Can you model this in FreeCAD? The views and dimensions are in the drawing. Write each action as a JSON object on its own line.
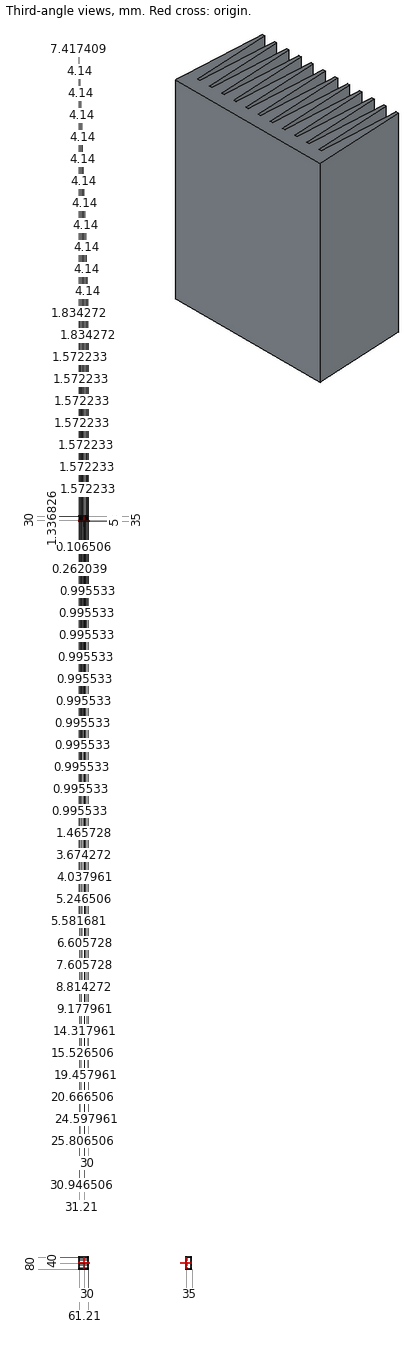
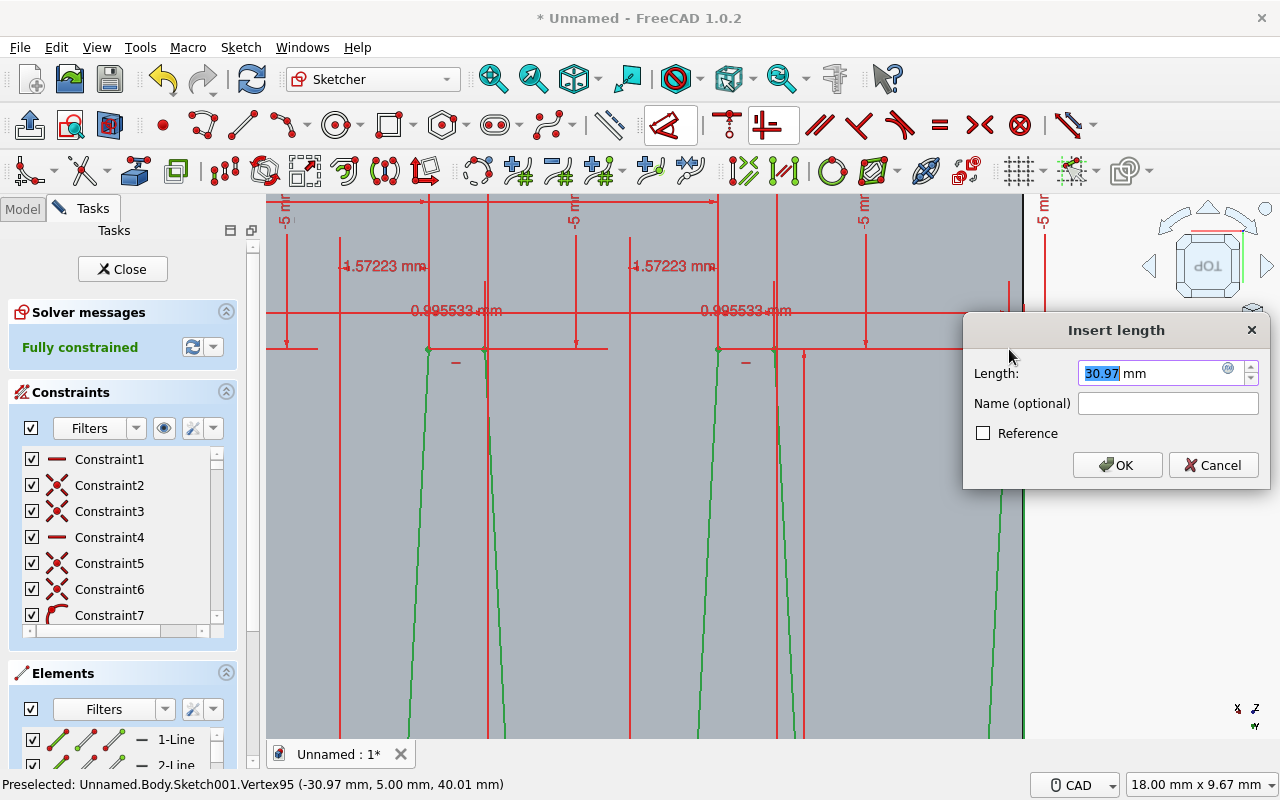
{"action": "type", "text": "30.946506"}
{"action": "key", "text": "Return"}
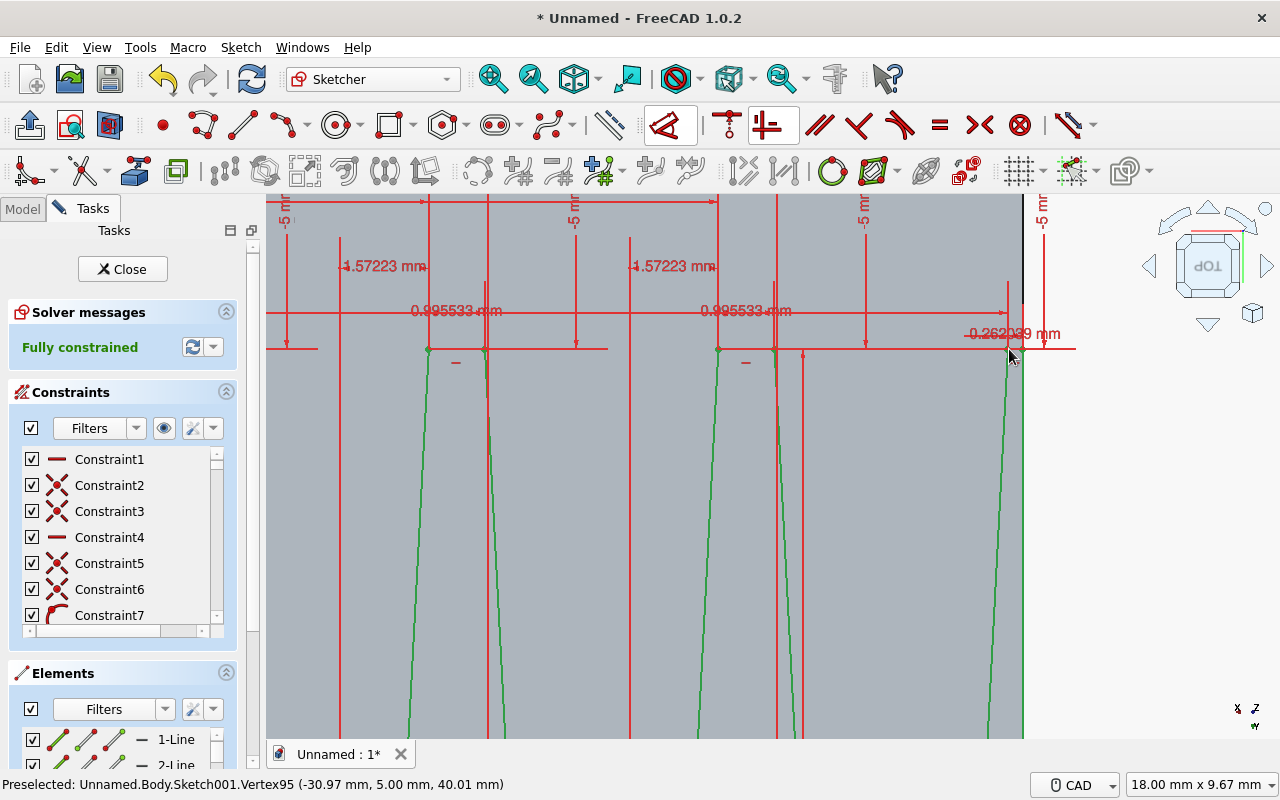
{"action": "left_click", "coordinate": [123, 269]}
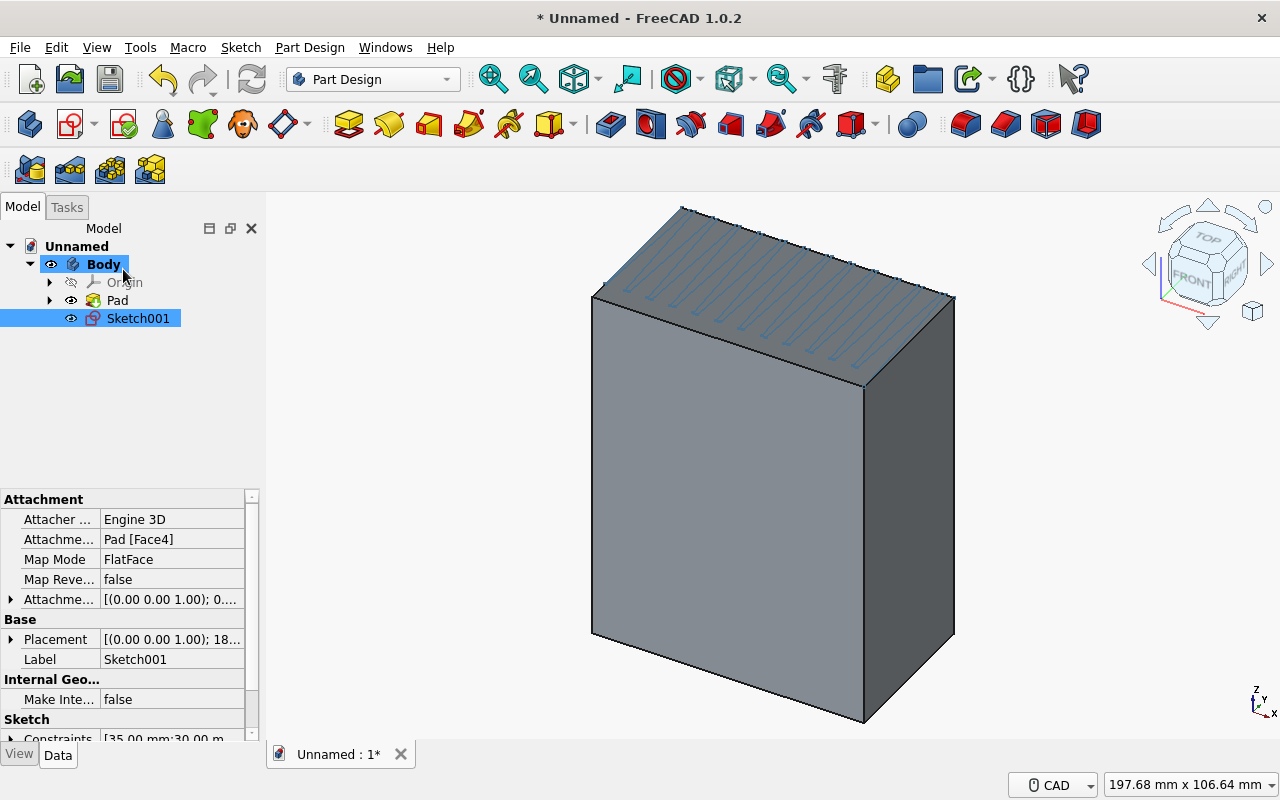
{"action": "left_click", "coordinate": [612, 124]}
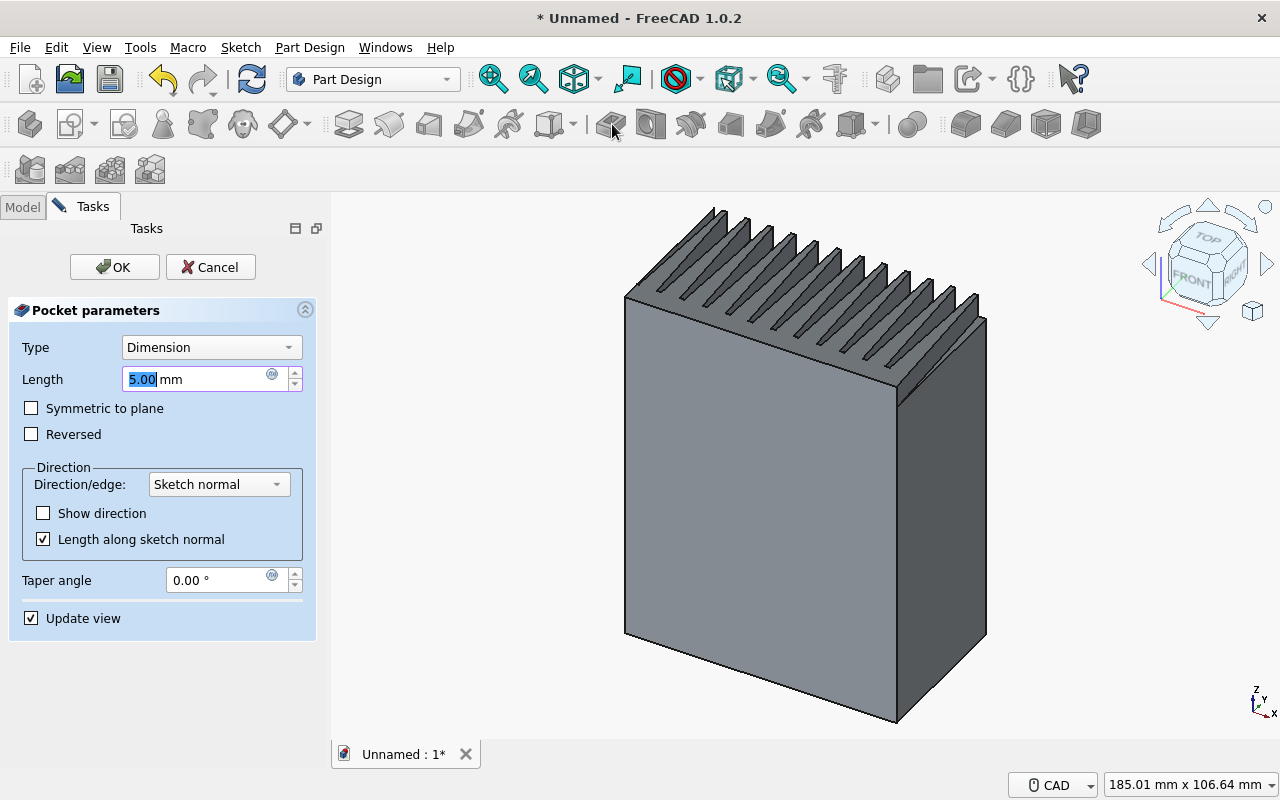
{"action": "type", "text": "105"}
{"action": "key", "text": "Tab"}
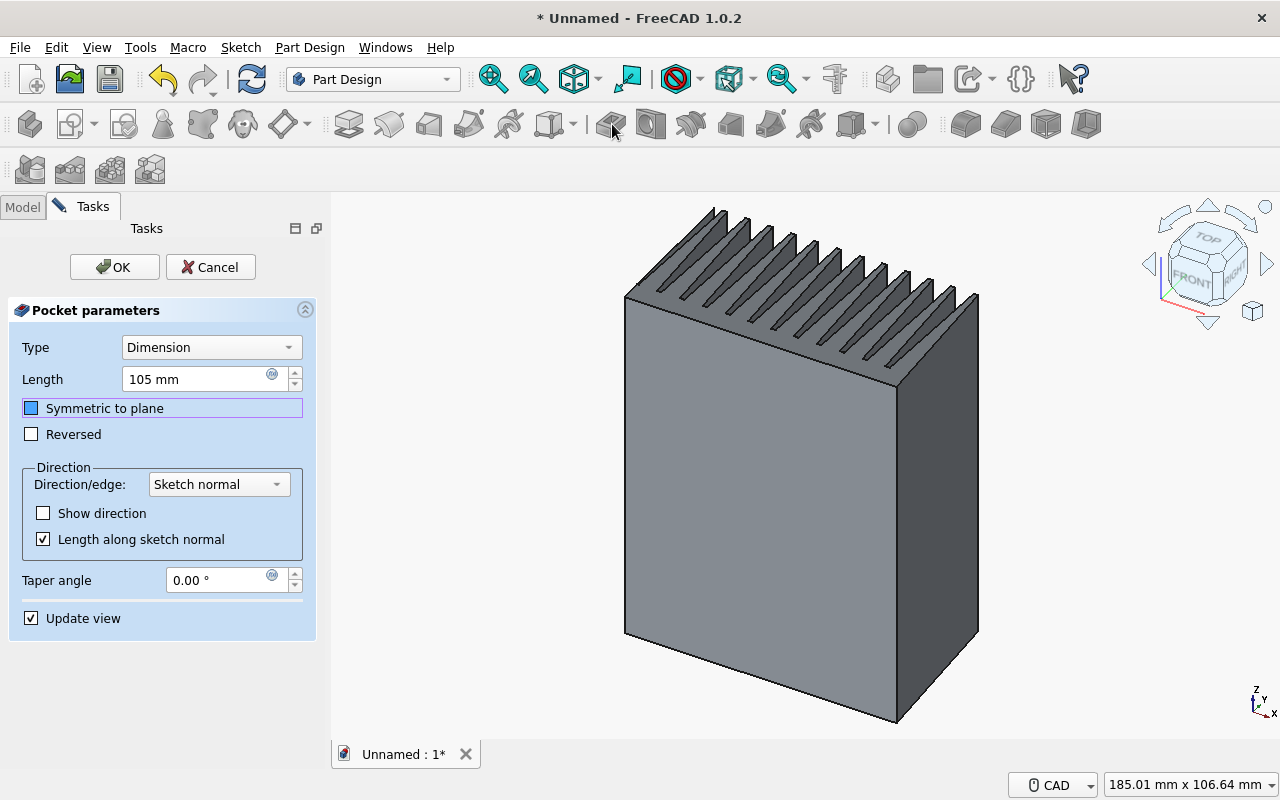
{"action": "left_click", "coordinate": [115, 267]}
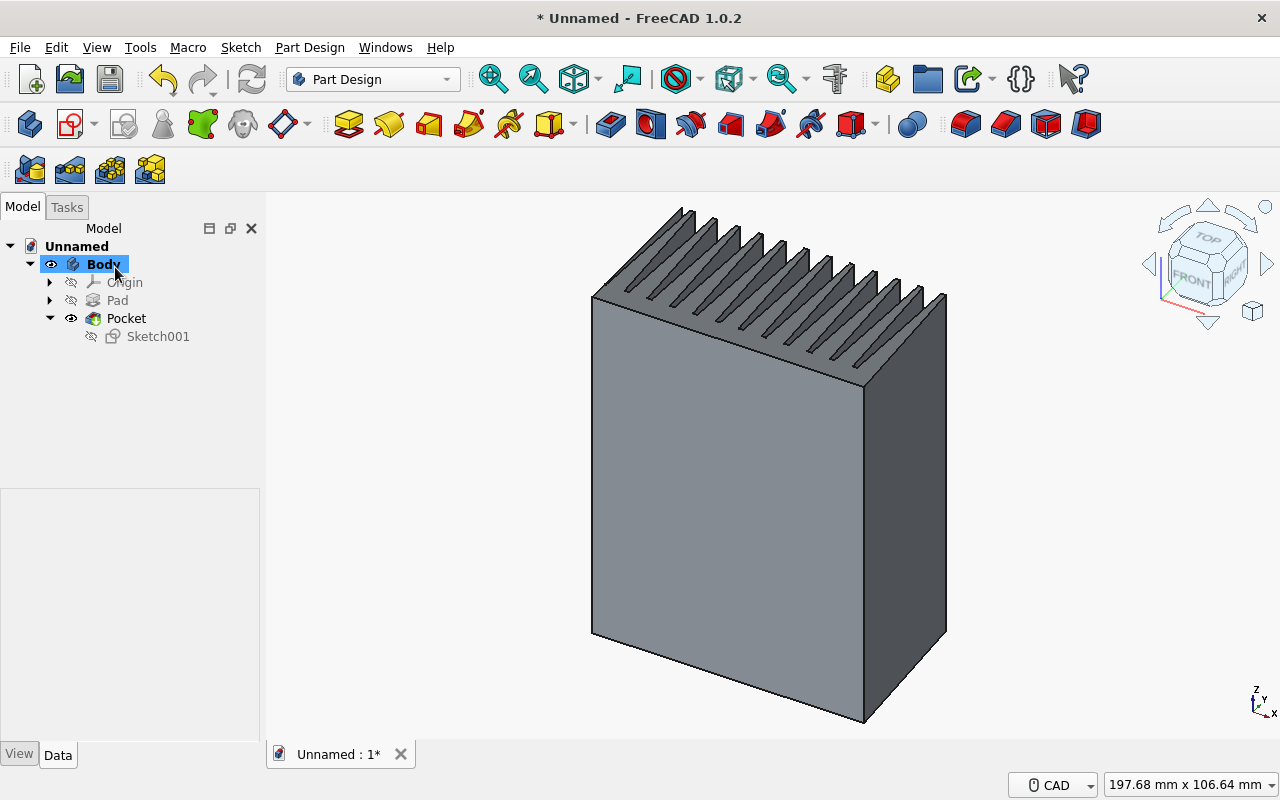
{"action": "key", "text": "0"}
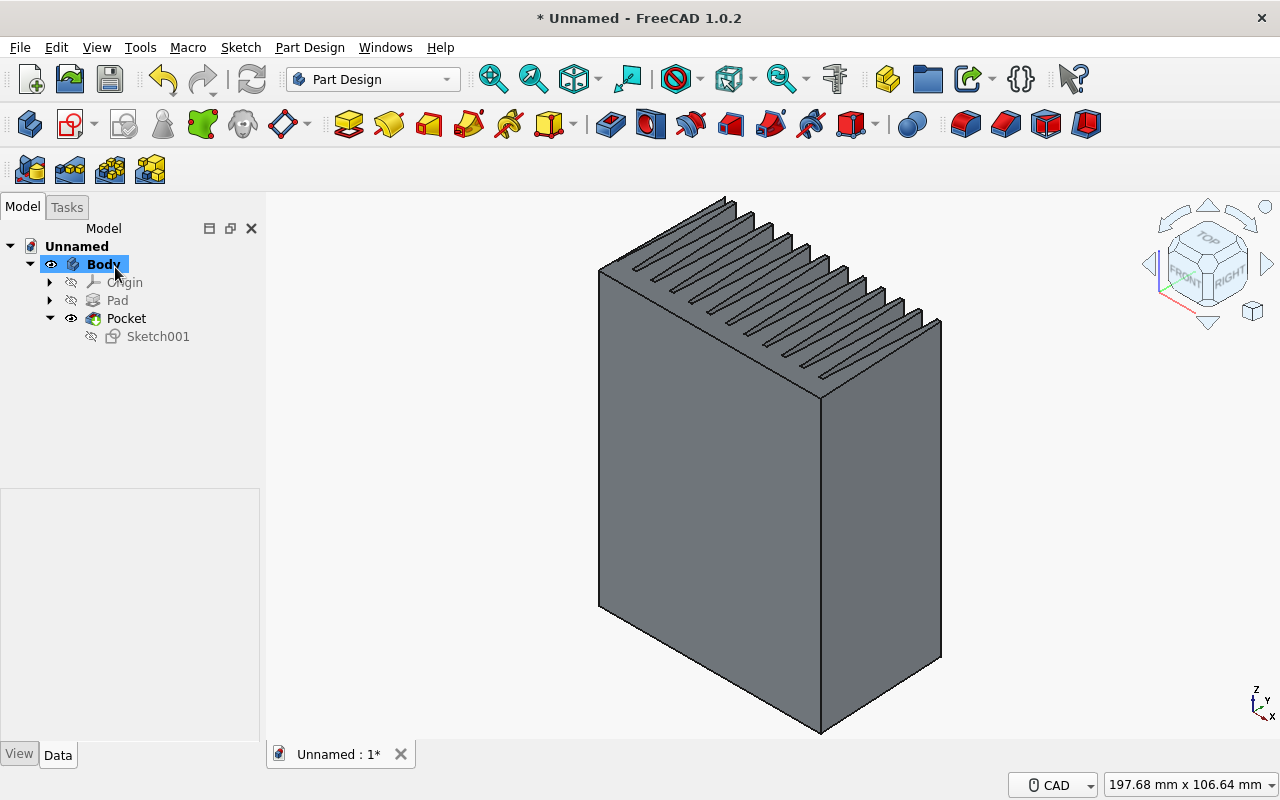
{"action": "left_click", "coordinate": [814, 383]}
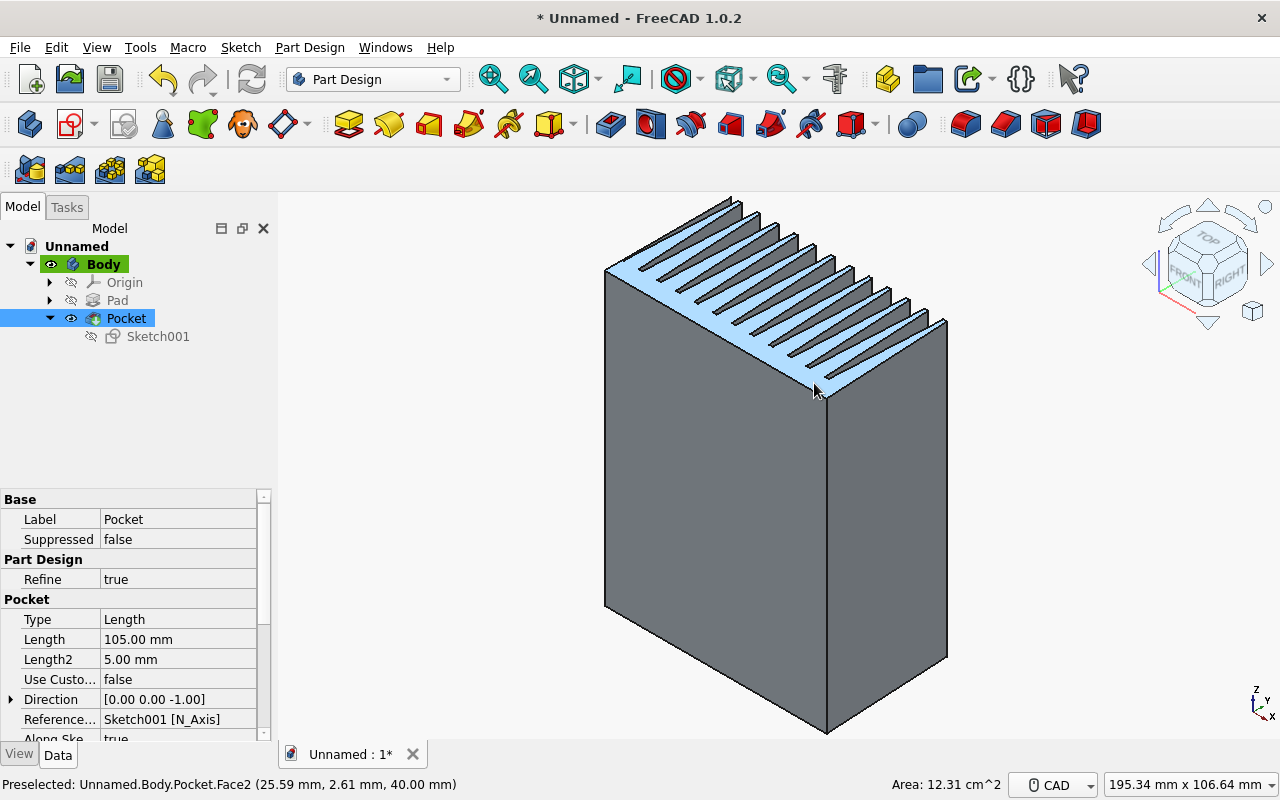
{"action": "left_click", "coordinate": [70, 124]}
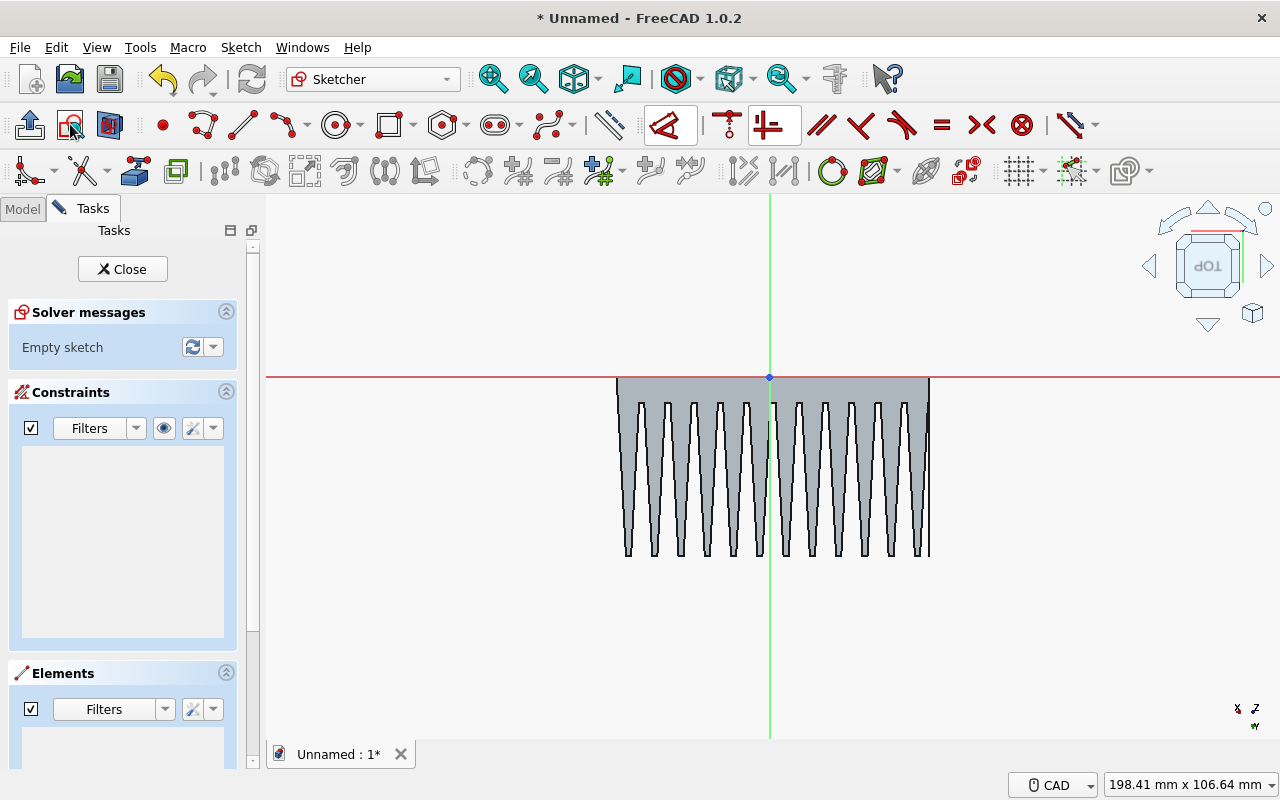
{"action": "scroll", "coordinate": [1058, 474], "scroll_direction": "up", "scroll_amount": 3}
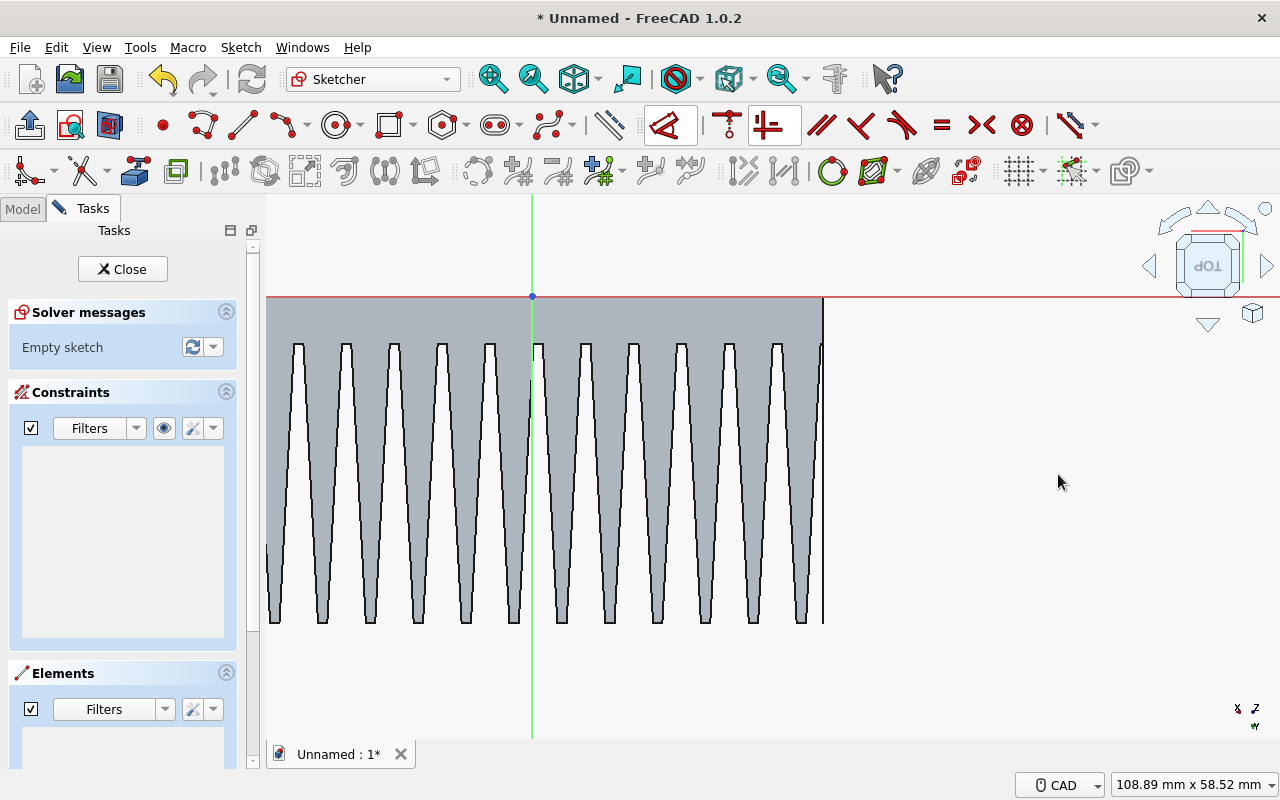
{"action": "key", "text": "g m"}